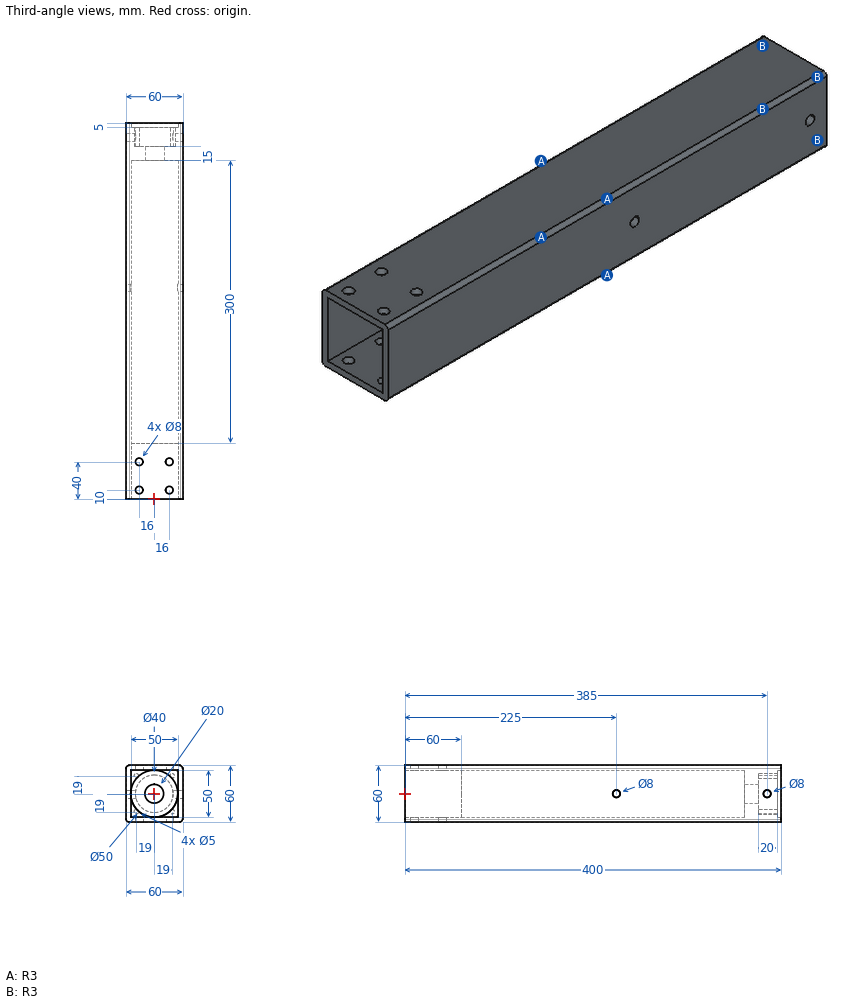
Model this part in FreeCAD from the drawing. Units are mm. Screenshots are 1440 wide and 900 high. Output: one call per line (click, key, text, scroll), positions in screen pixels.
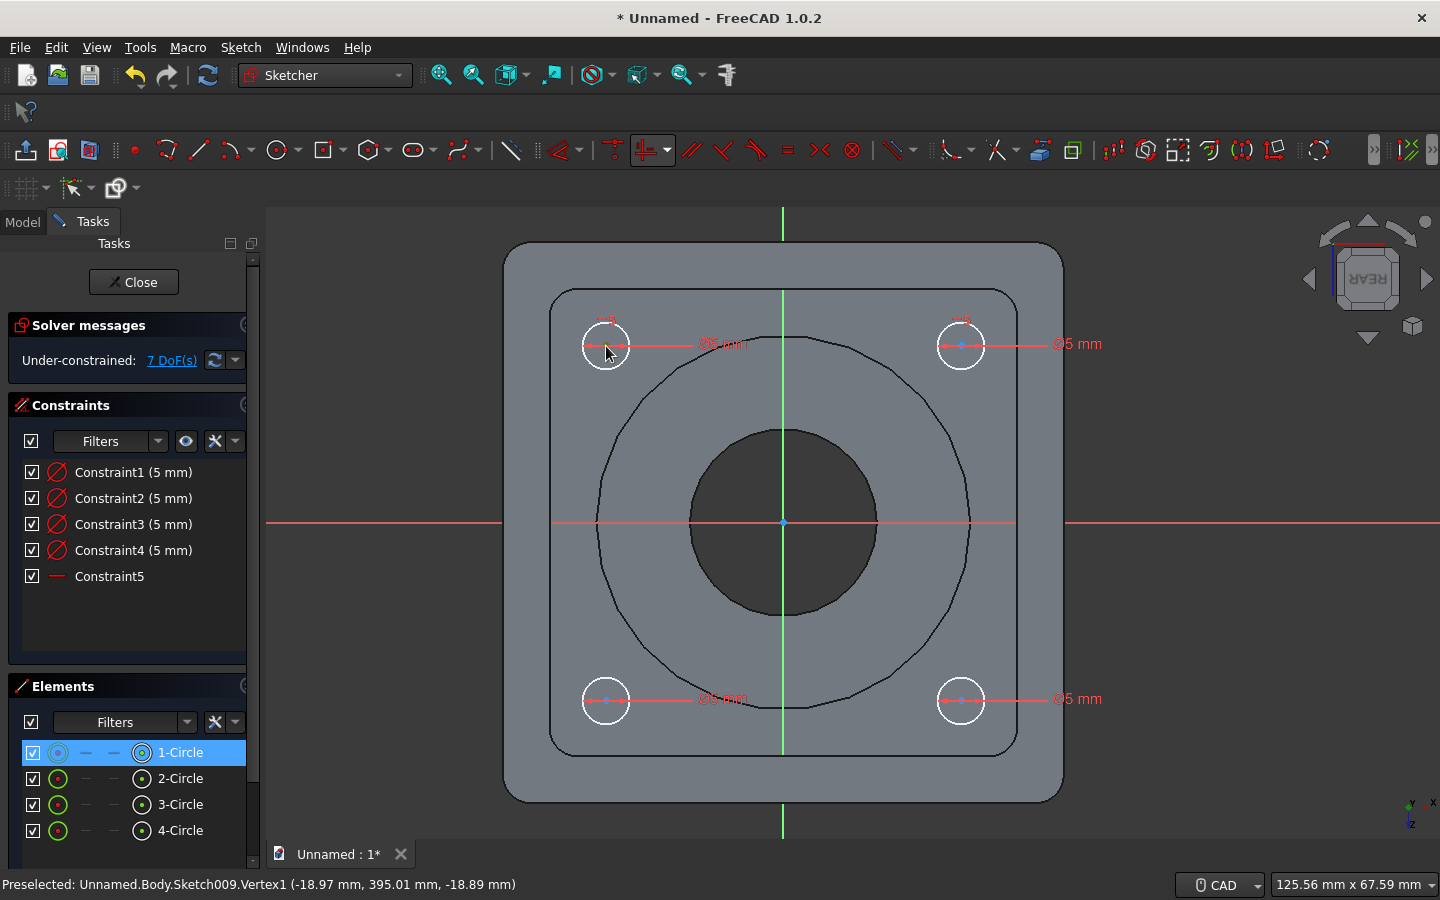
click(606, 701)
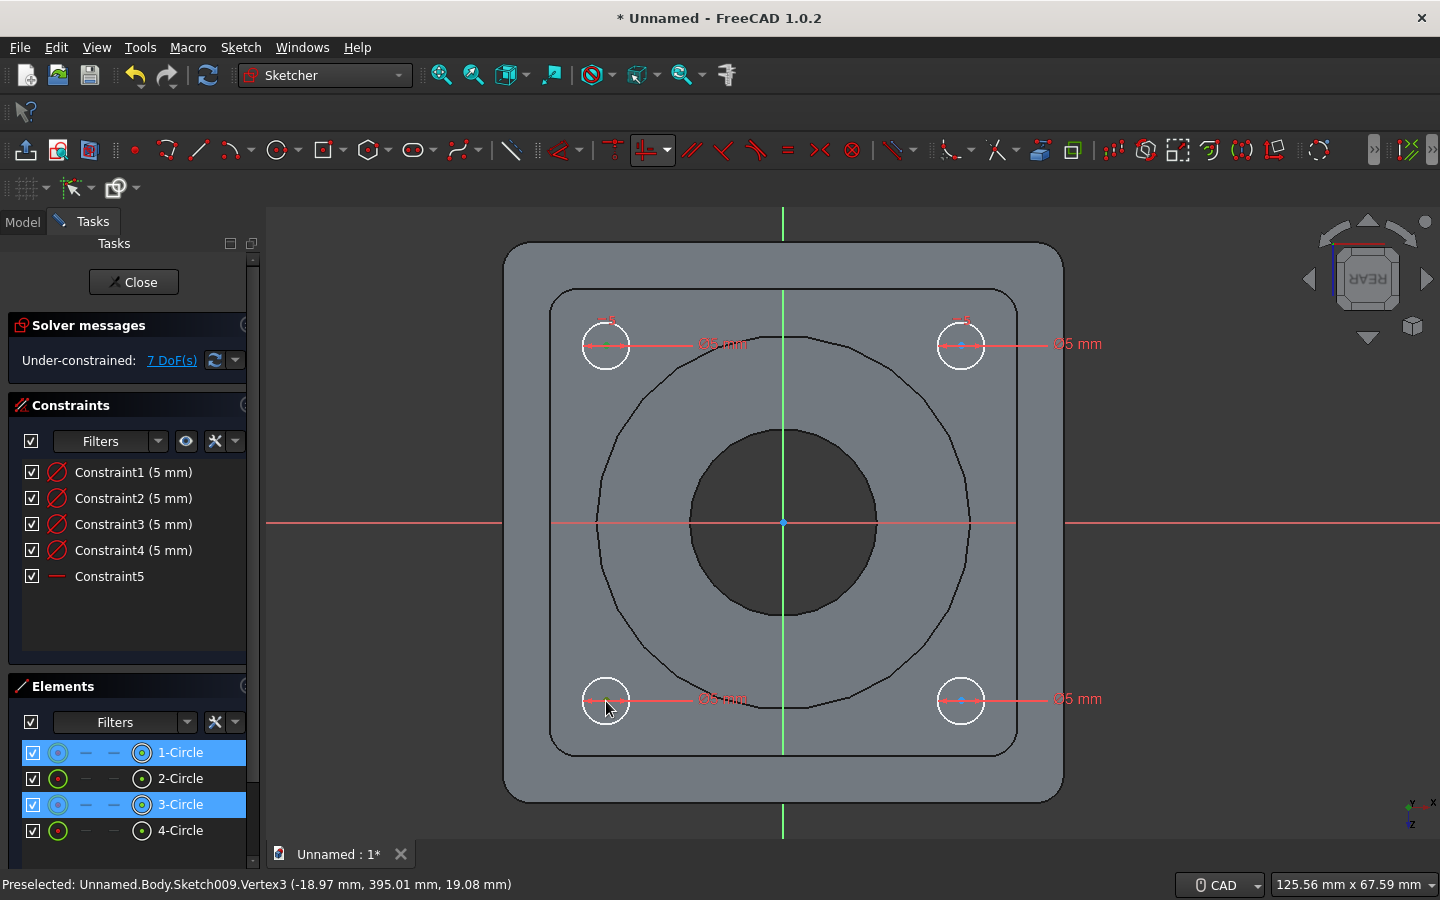
key(v)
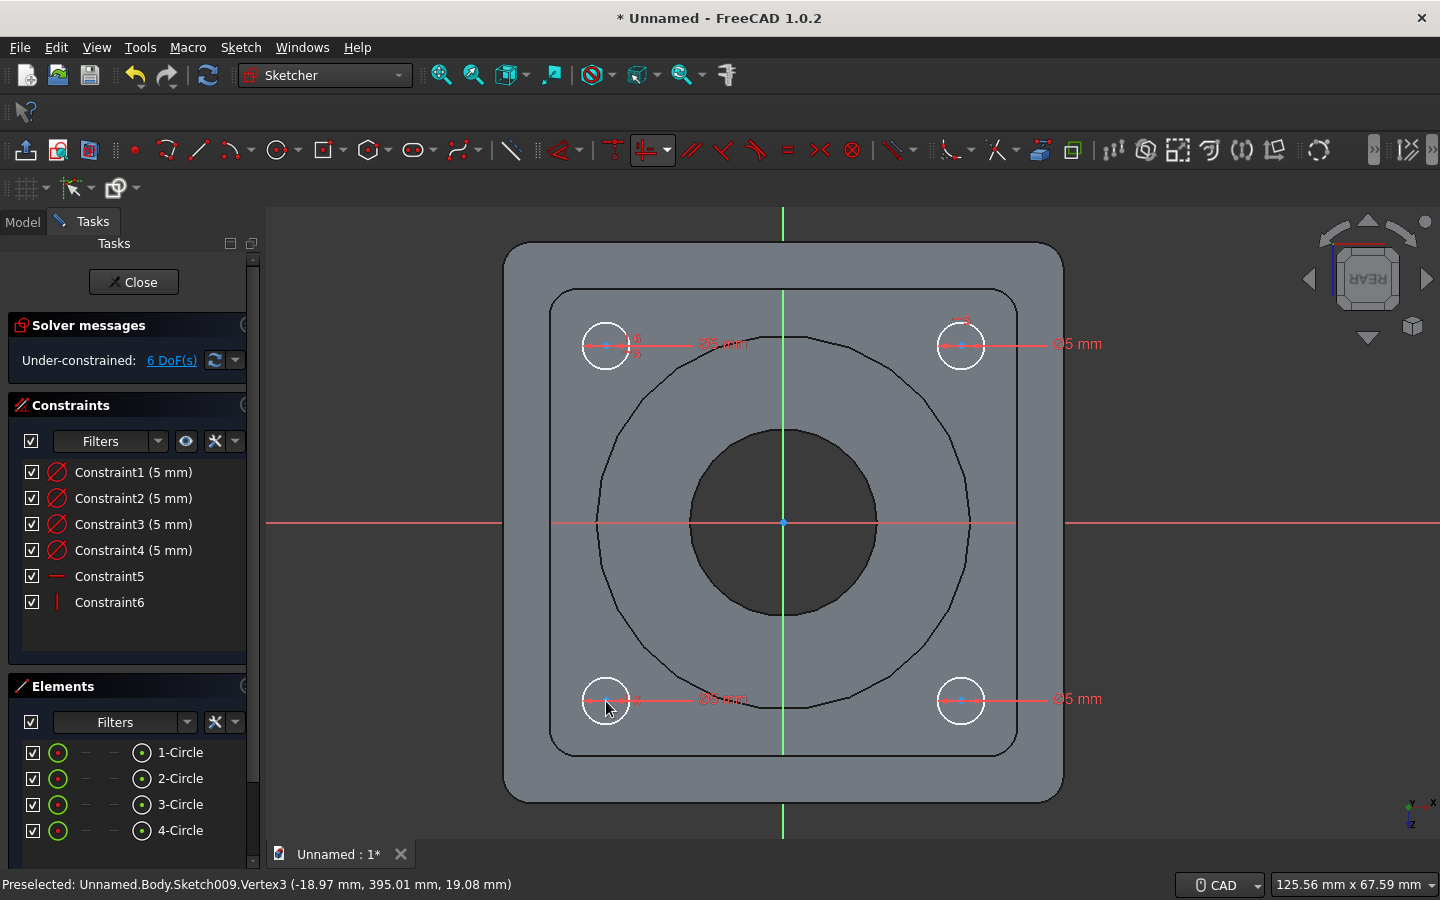
click(961, 346)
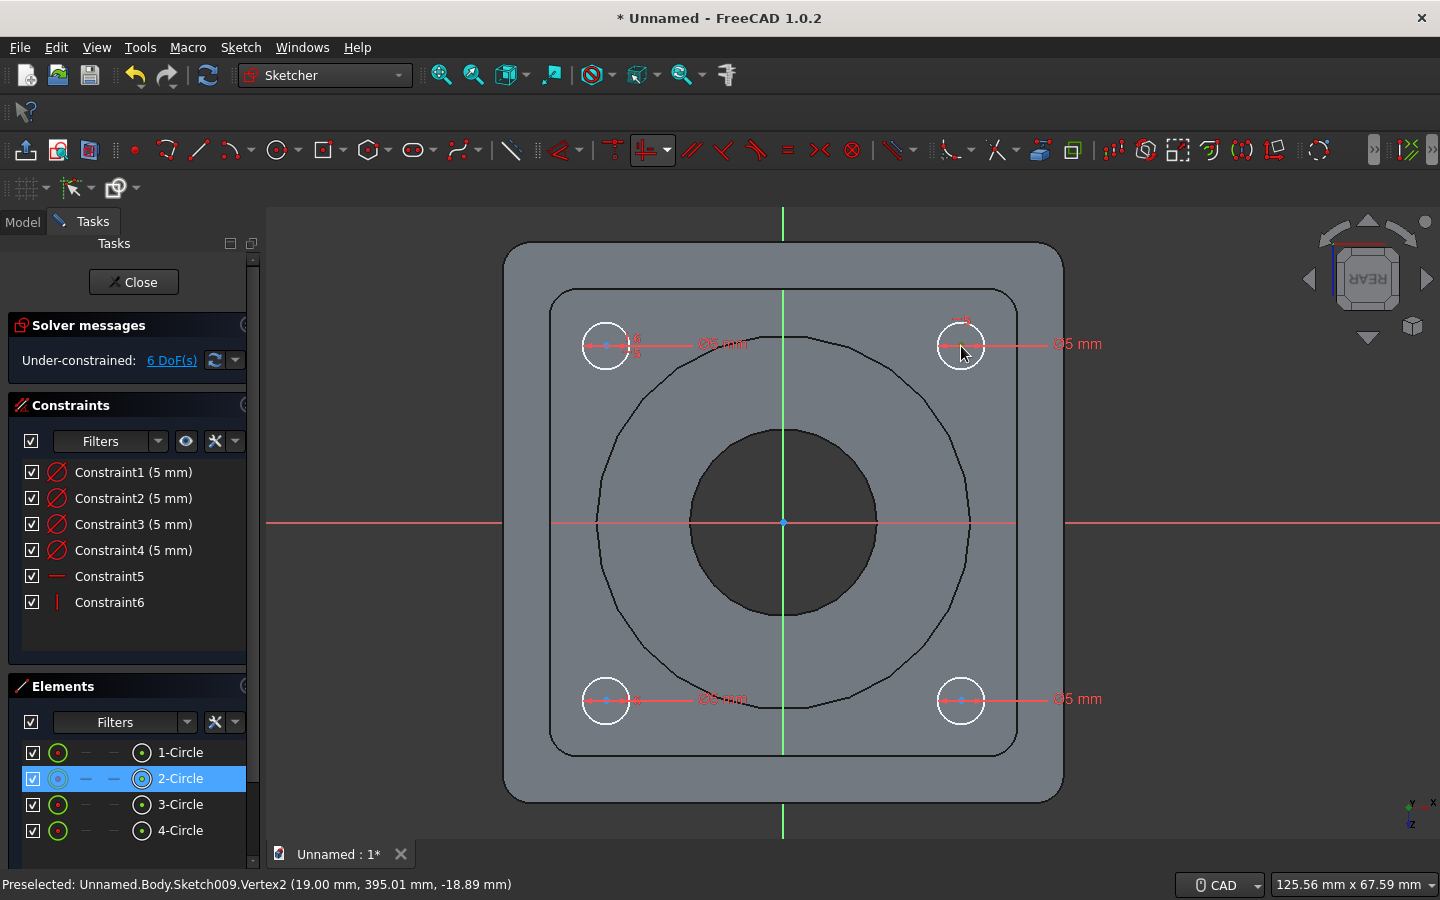
click(961, 701)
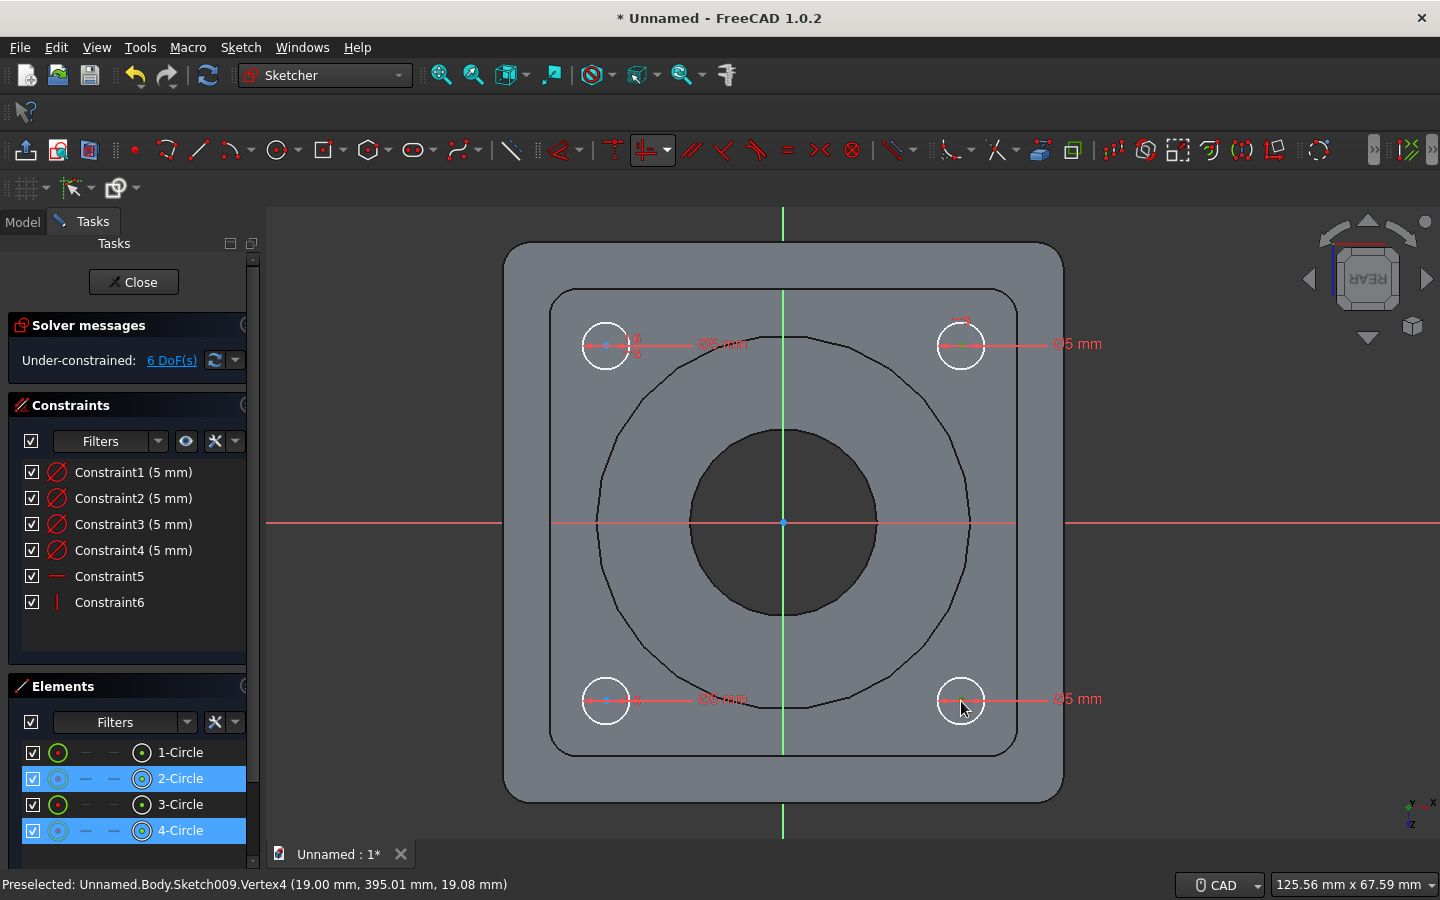
click(670, 150)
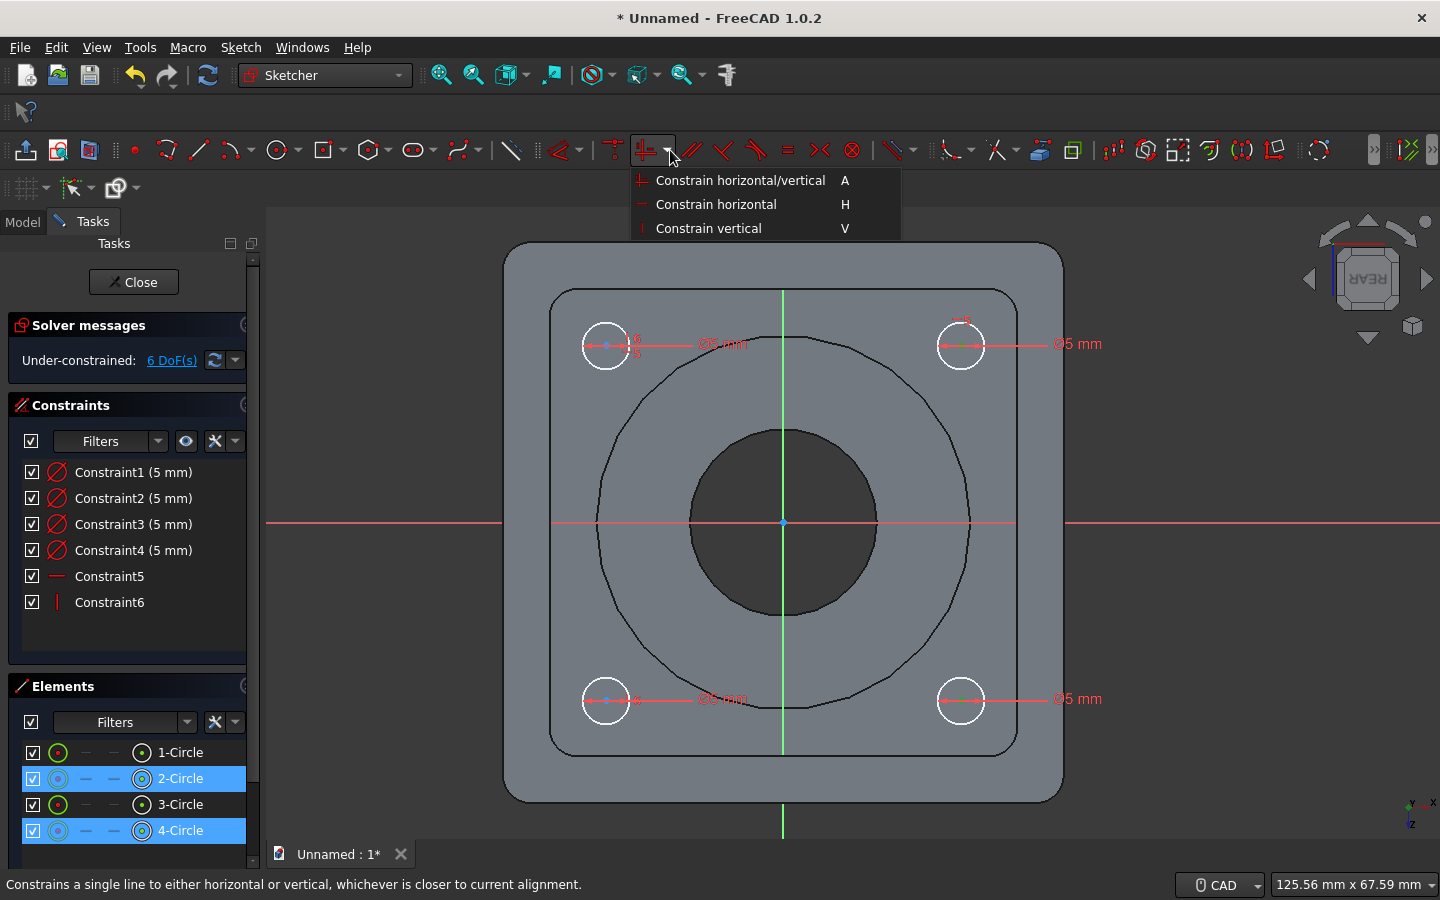
click(766, 228)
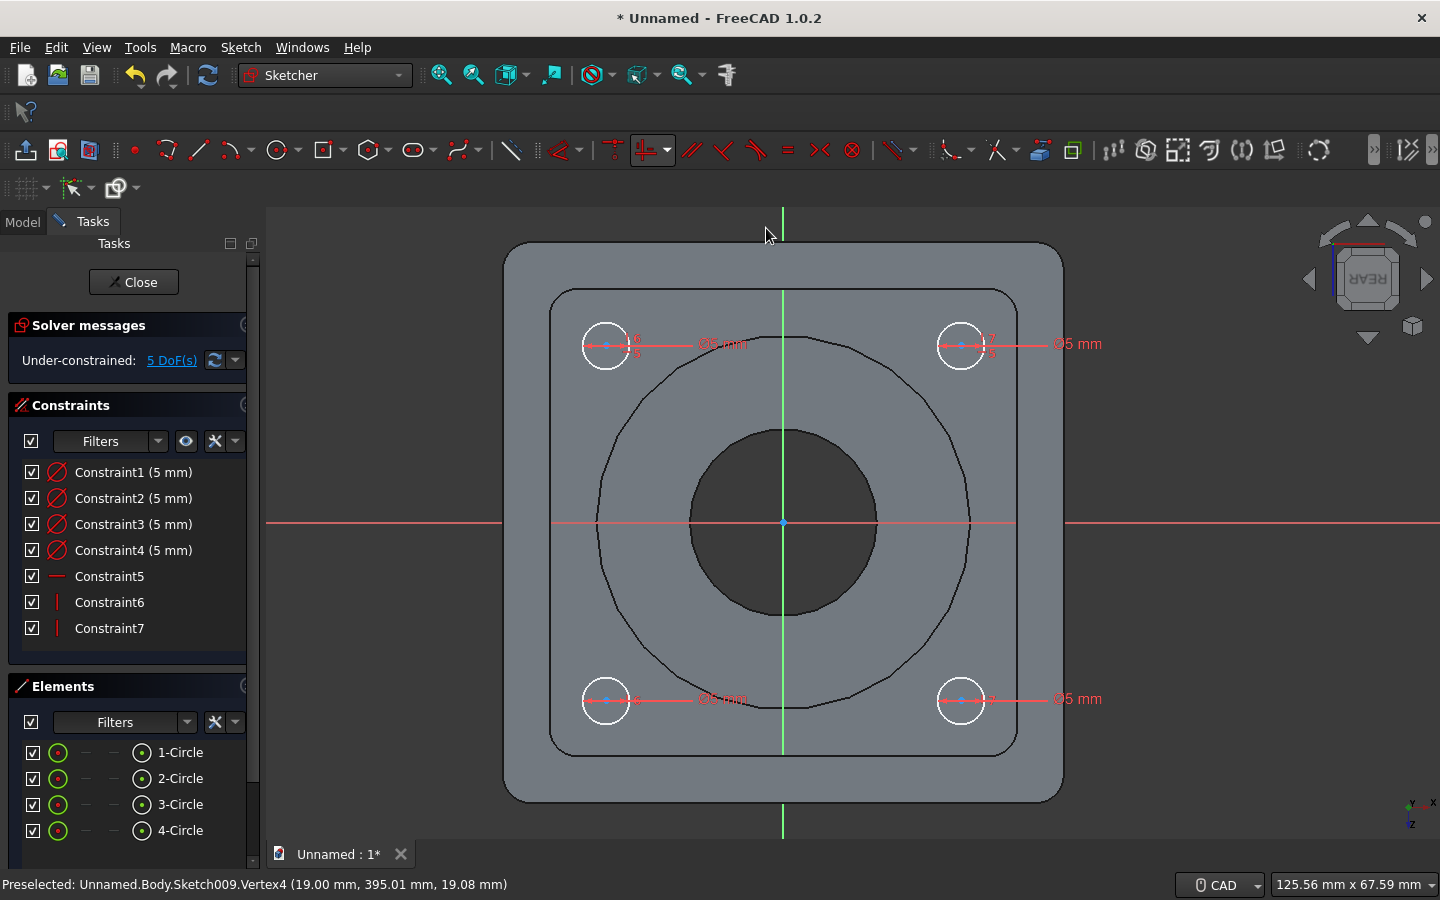
click(606, 701)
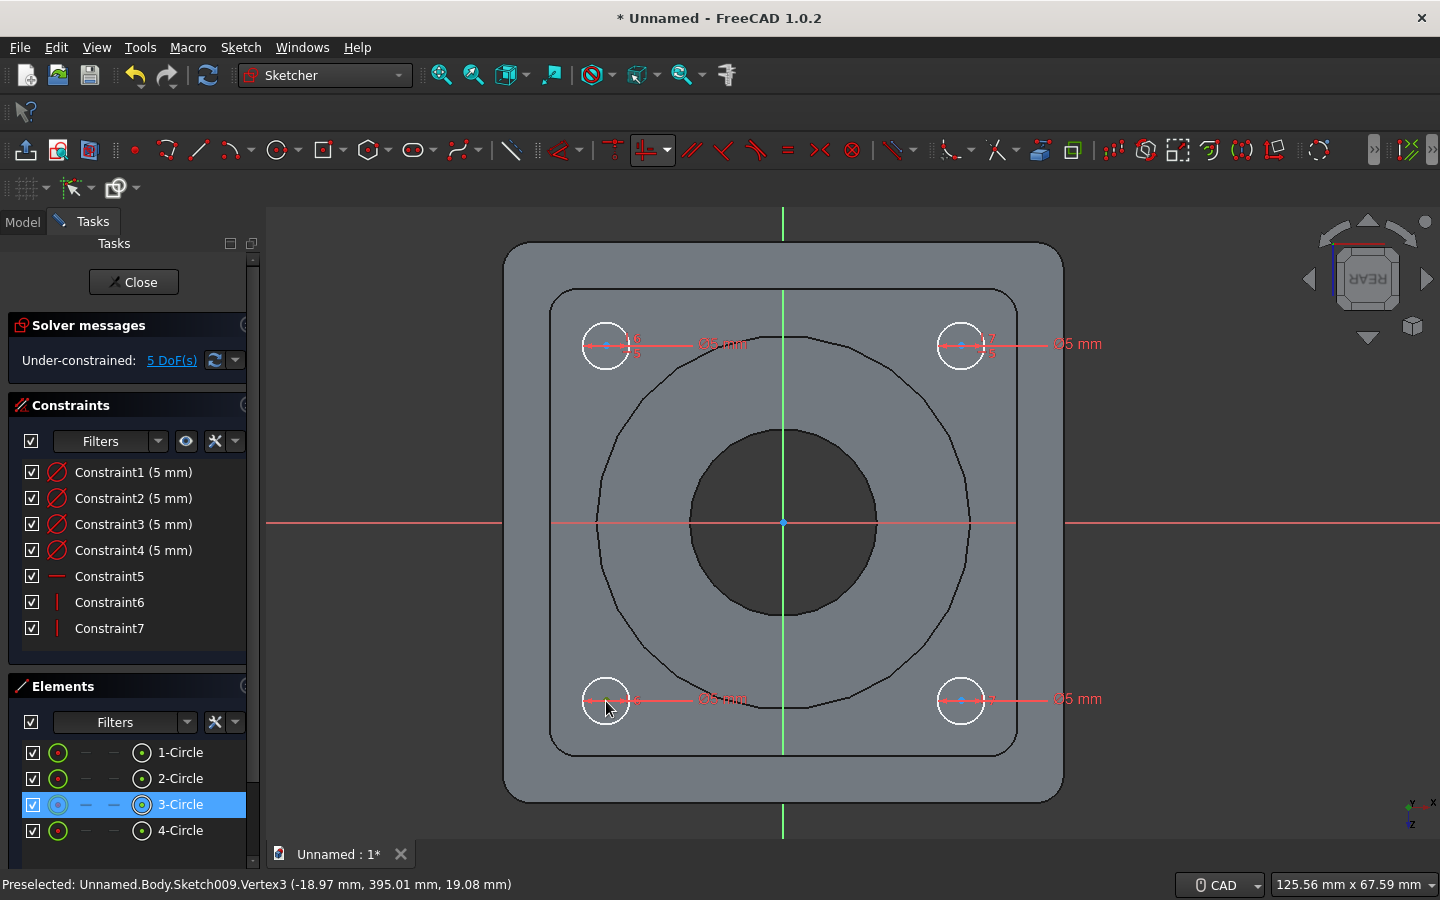
click(961, 701)